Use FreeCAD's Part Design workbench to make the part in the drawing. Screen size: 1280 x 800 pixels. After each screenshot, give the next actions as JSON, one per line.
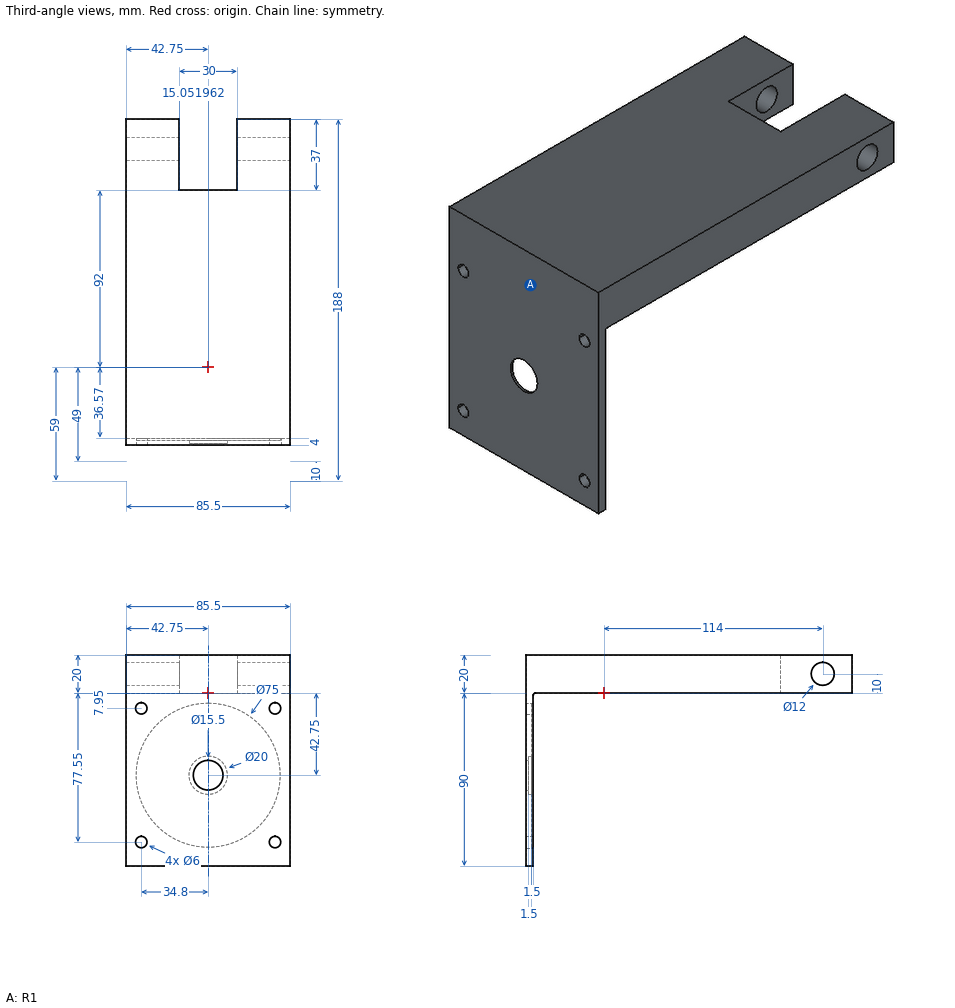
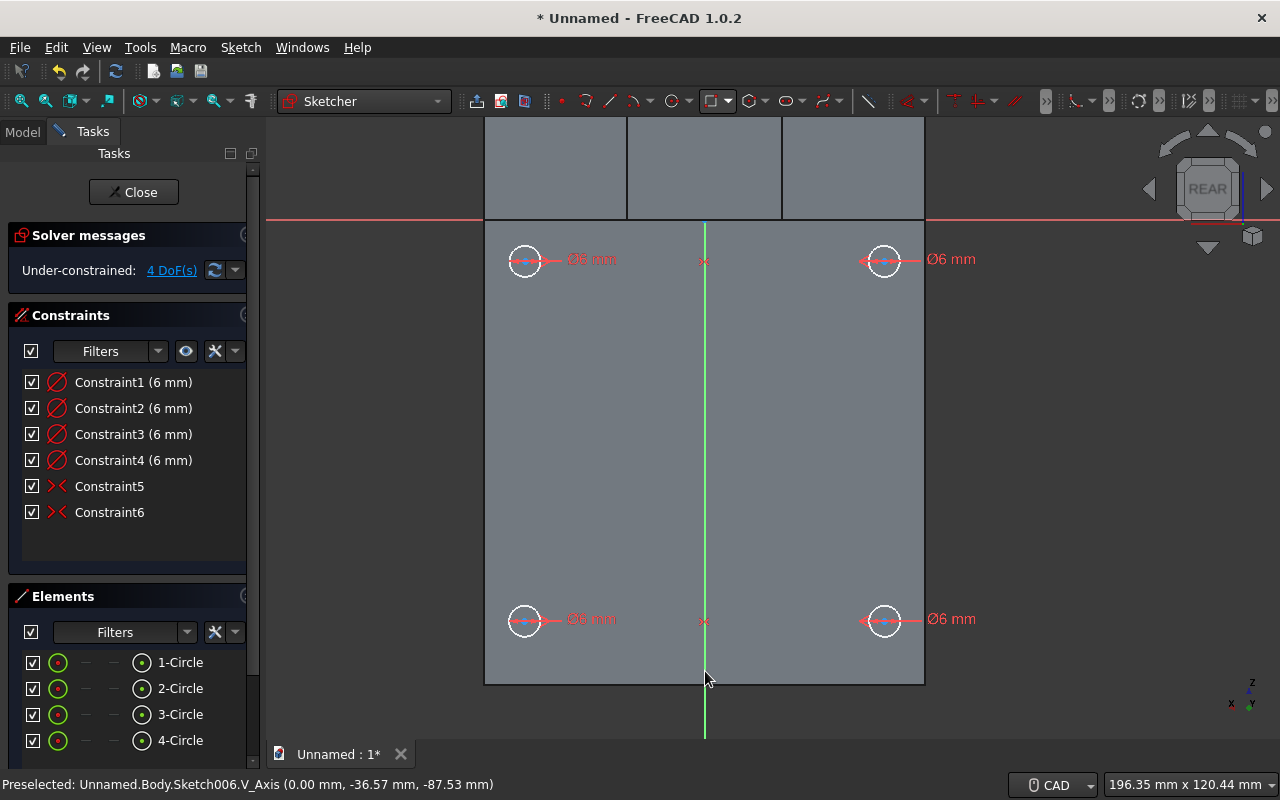
{"action": "left_click", "coordinate": [908, 102]}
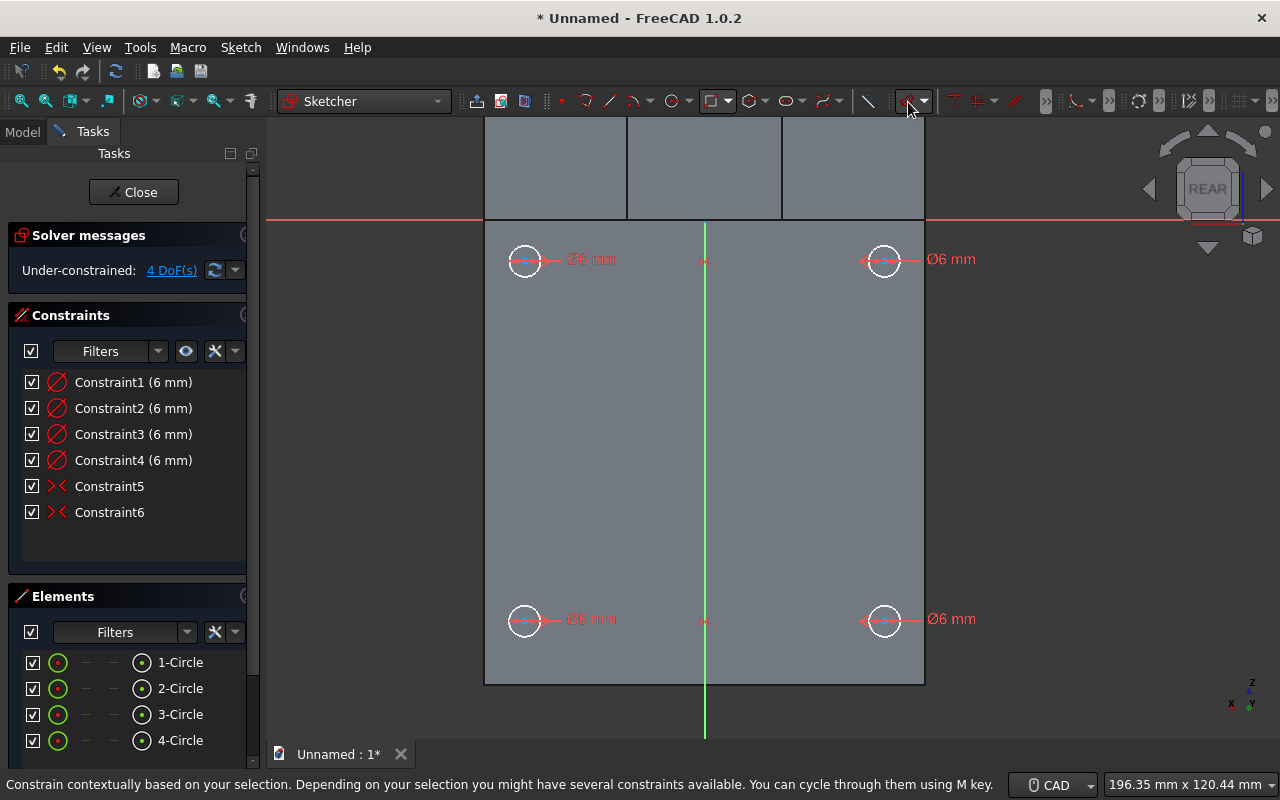
{"action": "left_click", "coordinate": [885, 621]}
{"action": "left_click", "coordinate": [795, 186]}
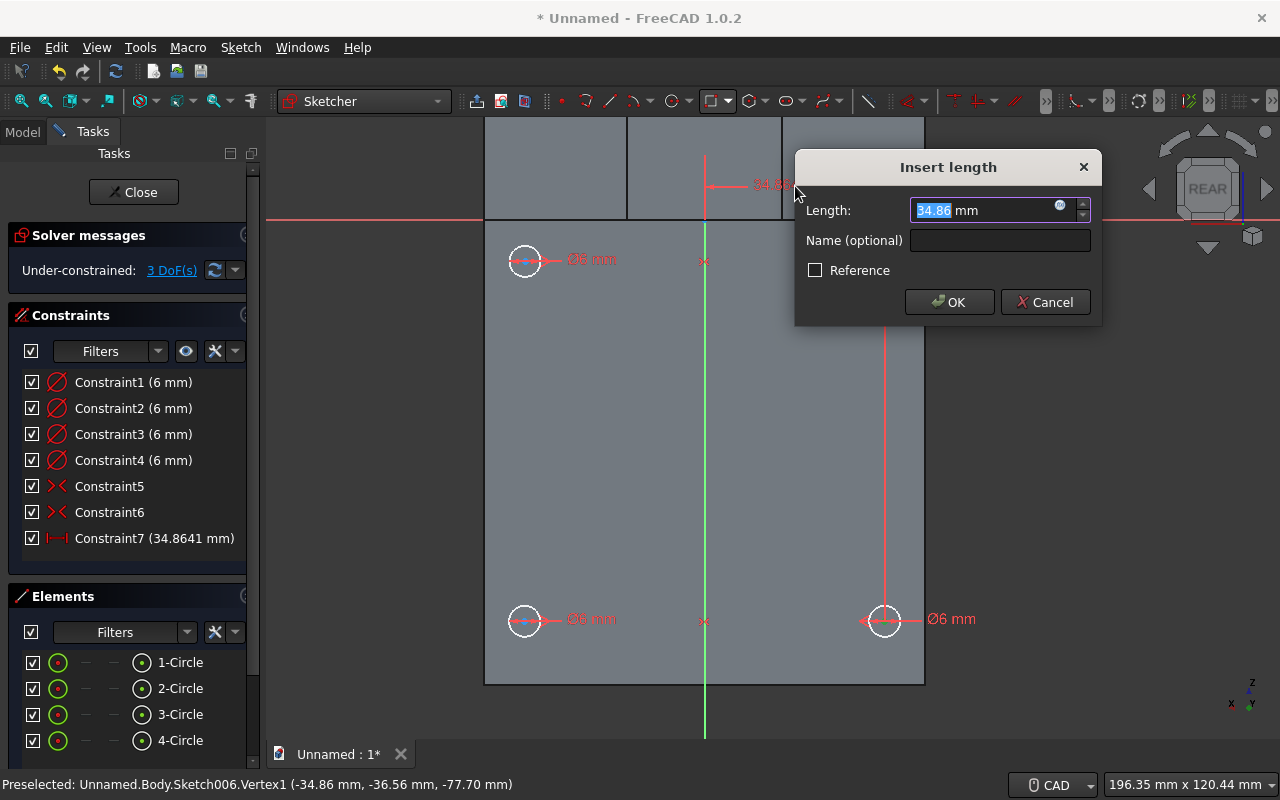
{"action": "type", "text": "34.8"}
{"action": "key", "text": "Return"}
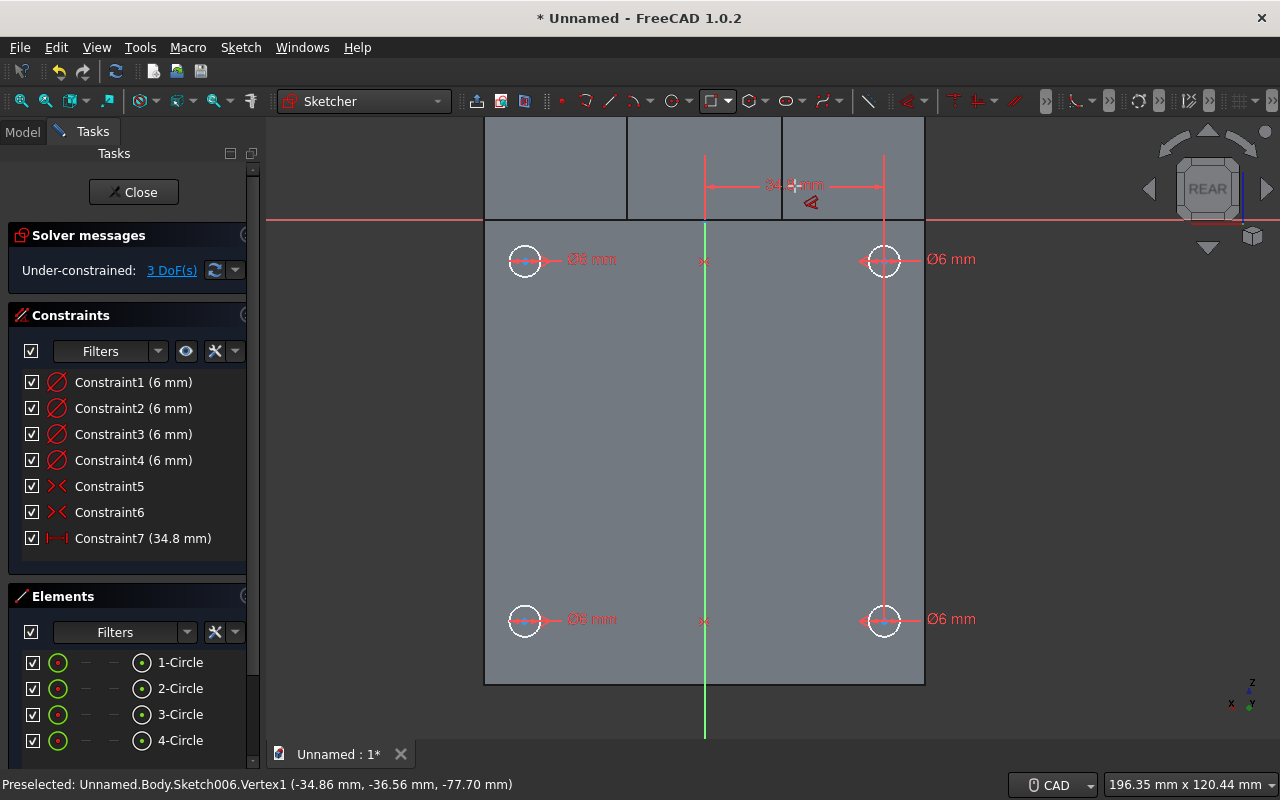
{"action": "left_click", "coordinate": [884, 261]}
{"action": "left_click", "coordinate": [794, 295]}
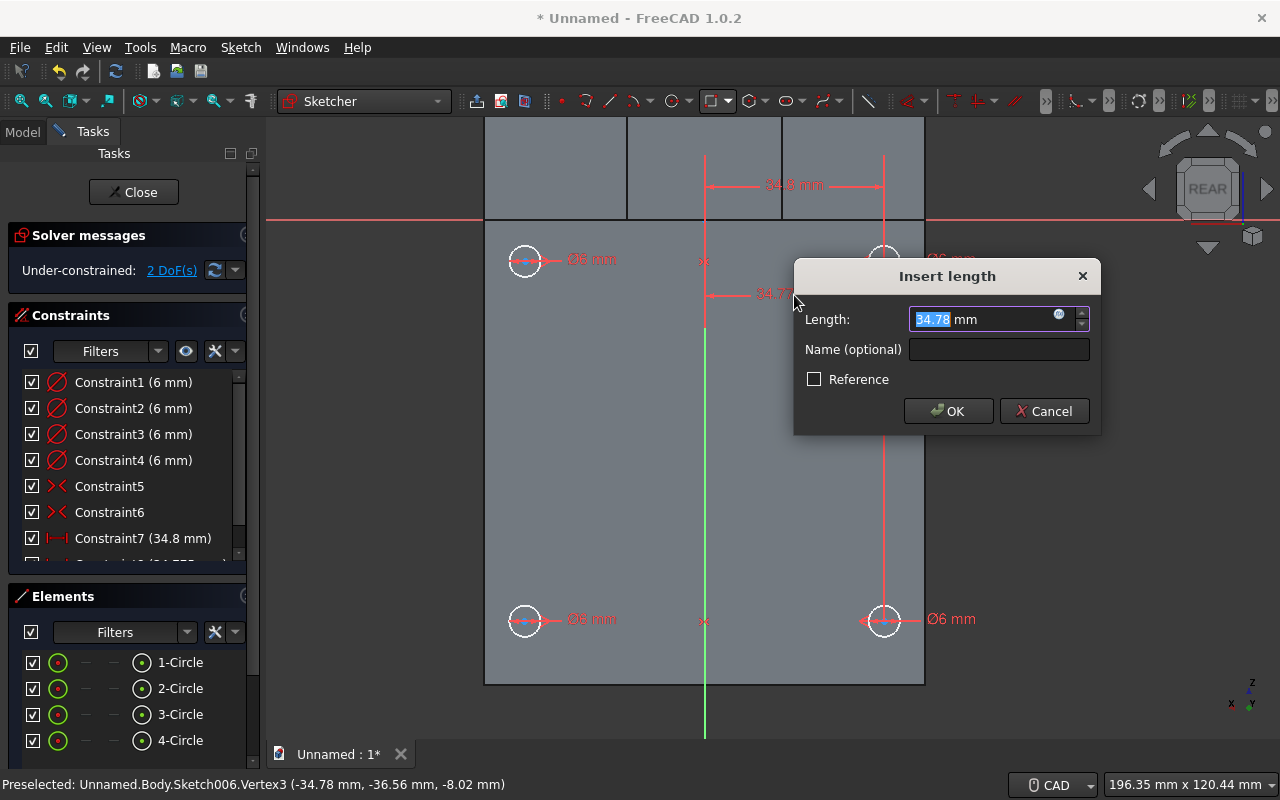
{"action": "type", "text": "34.8"}
{"action": "key", "text": "Return"}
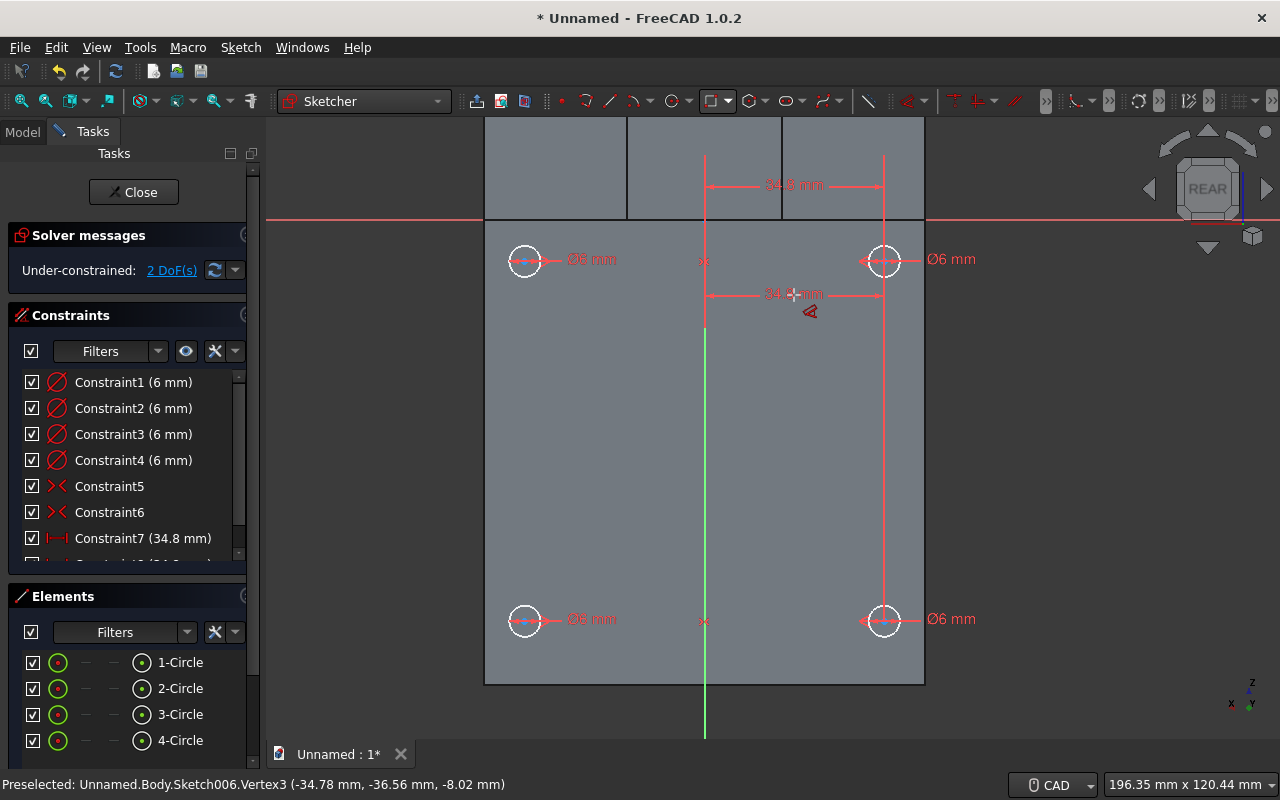
{"action": "left_click", "coordinate": [884, 261]}
{"action": "left_click", "coordinate": [918, 241]}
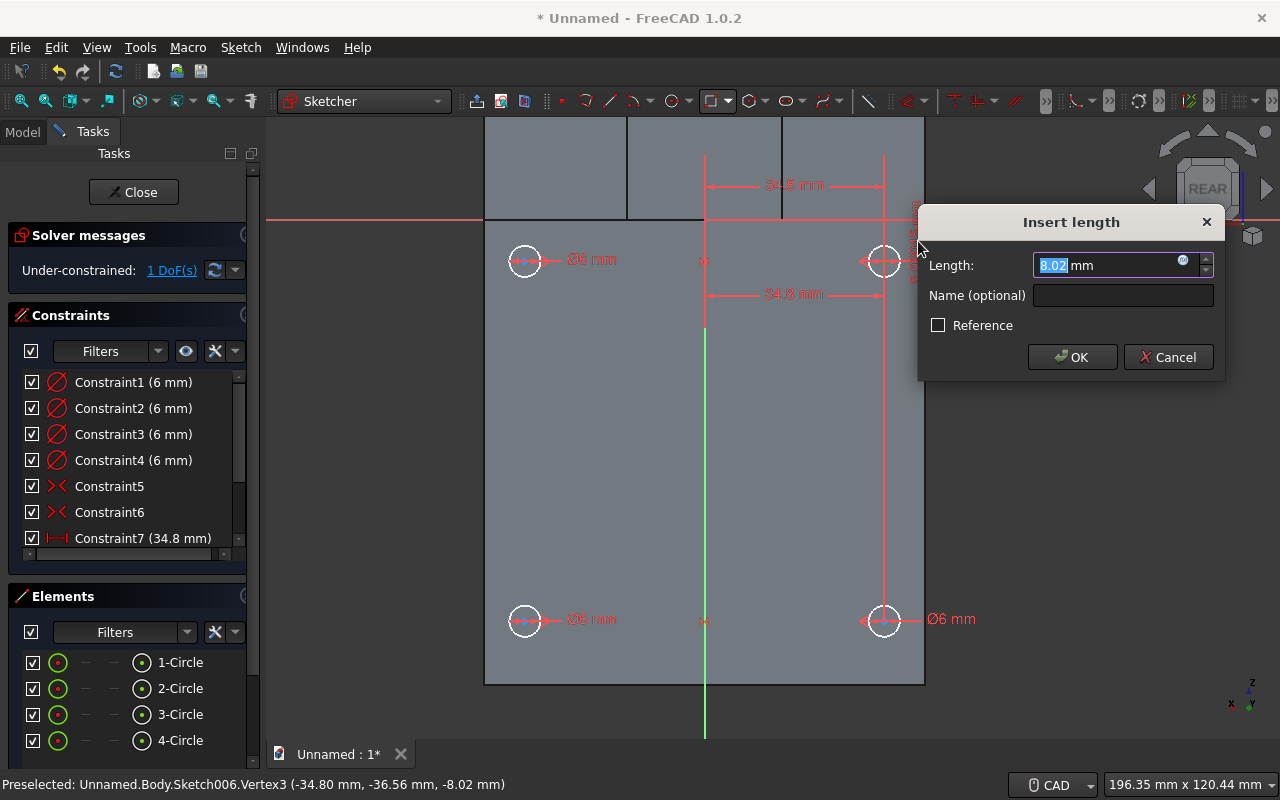
{"action": "type", "text": "7.95"}
{"action": "key", "text": "Return"}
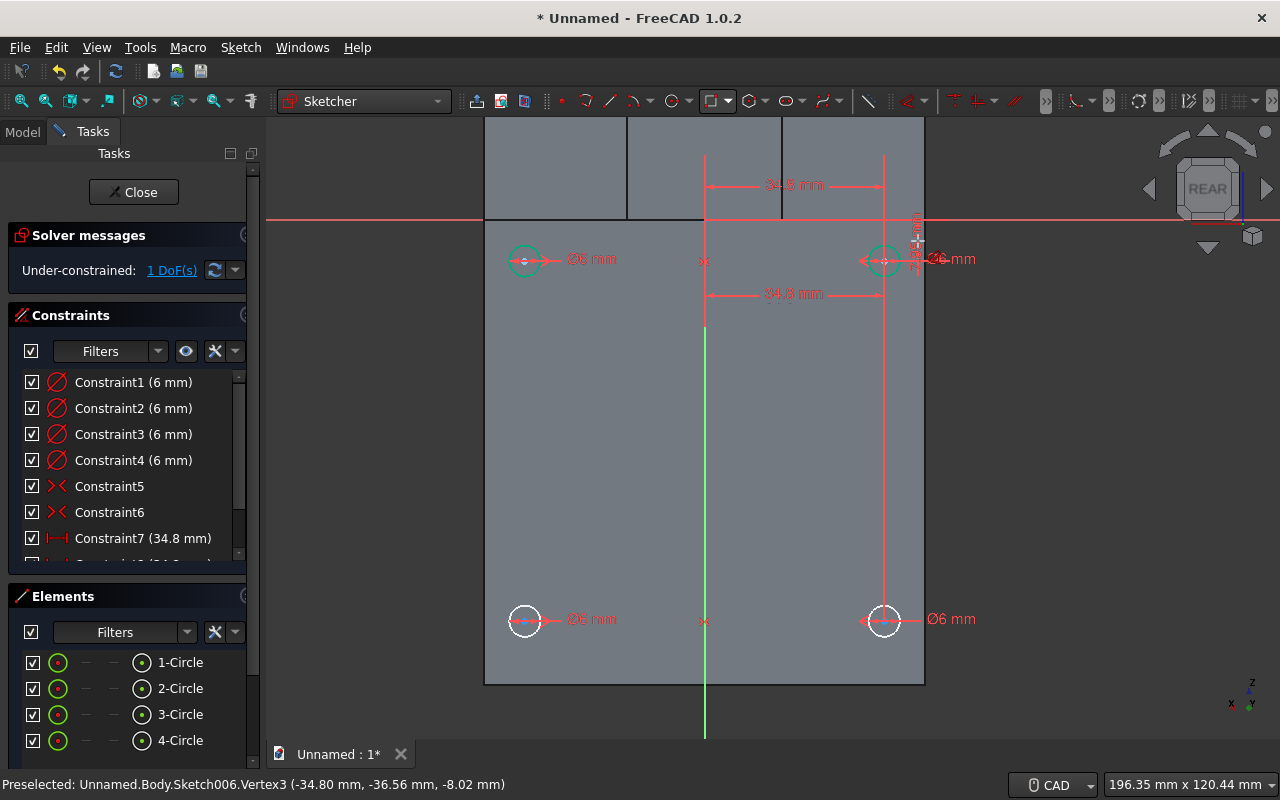
{"action": "left_click", "coordinate": [884, 621]}
{"action": "left_click", "coordinate": [918, 421]}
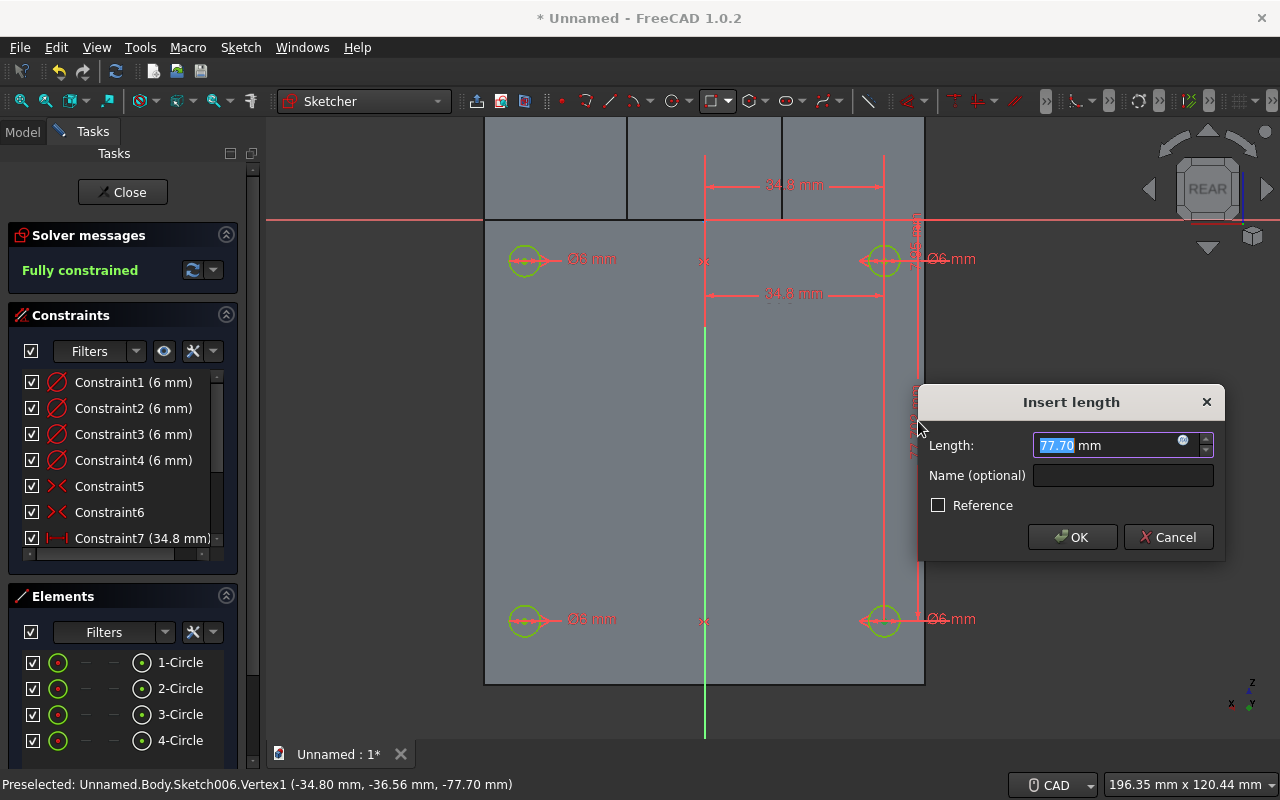
{"action": "type", "text": "77.55"}
{"action": "key", "text": "Return"}
{"action": "key", "text": "Escape"}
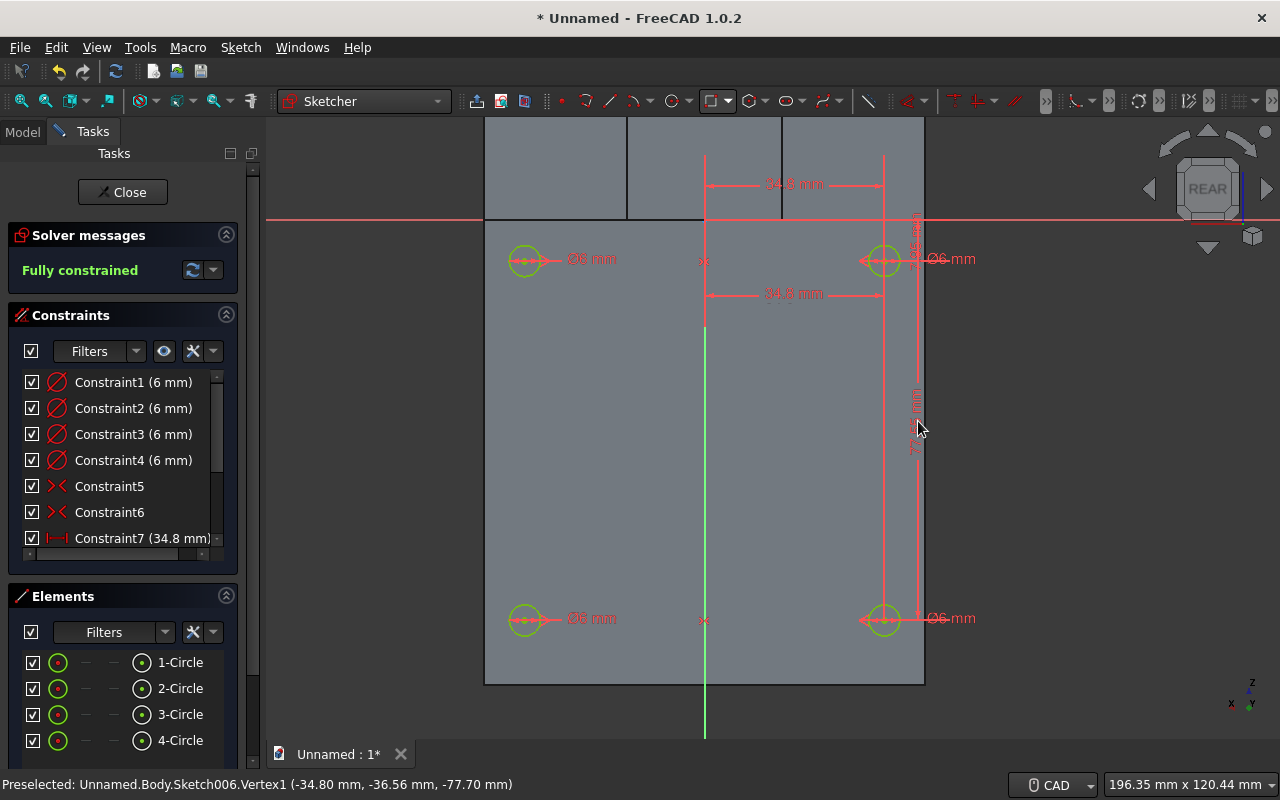
{"action": "left_click", "coordinate": [123, 192]}